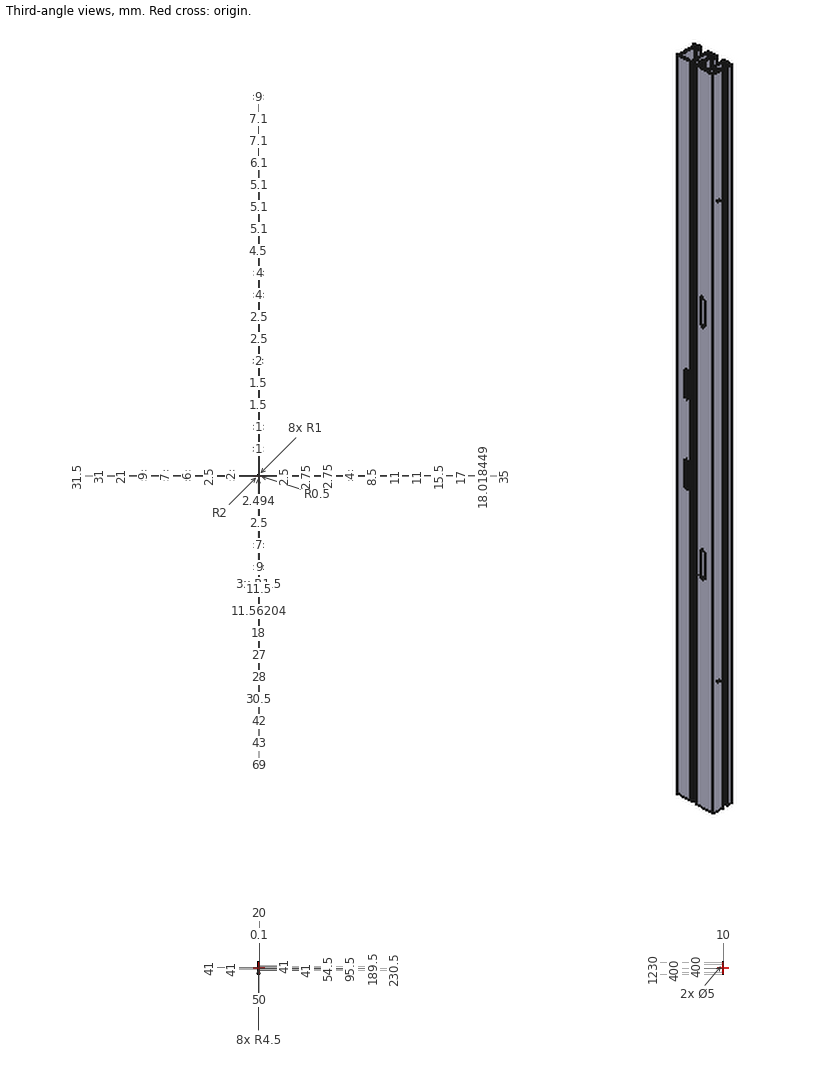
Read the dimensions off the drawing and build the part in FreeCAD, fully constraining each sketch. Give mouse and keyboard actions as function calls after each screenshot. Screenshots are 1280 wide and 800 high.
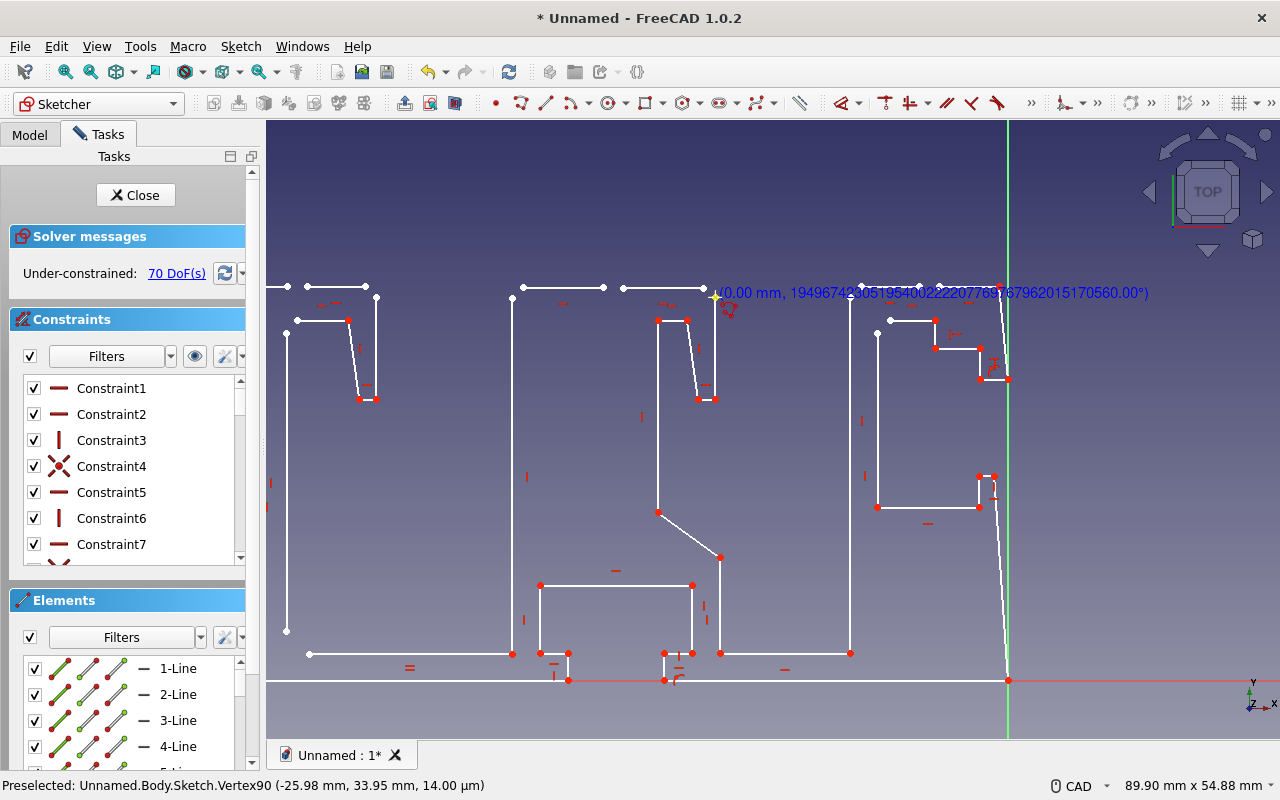
key(g)
key(3)
key(a)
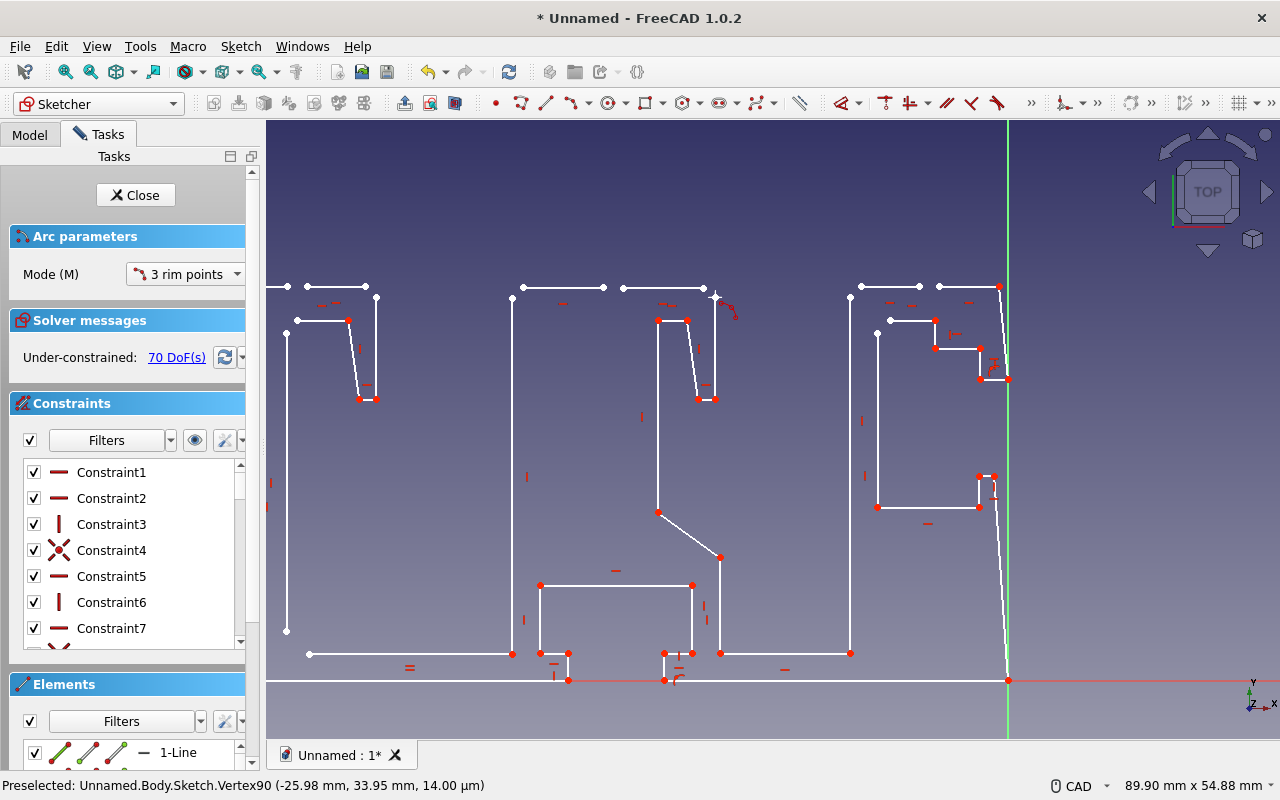
click(624, 288)
click(604, 288)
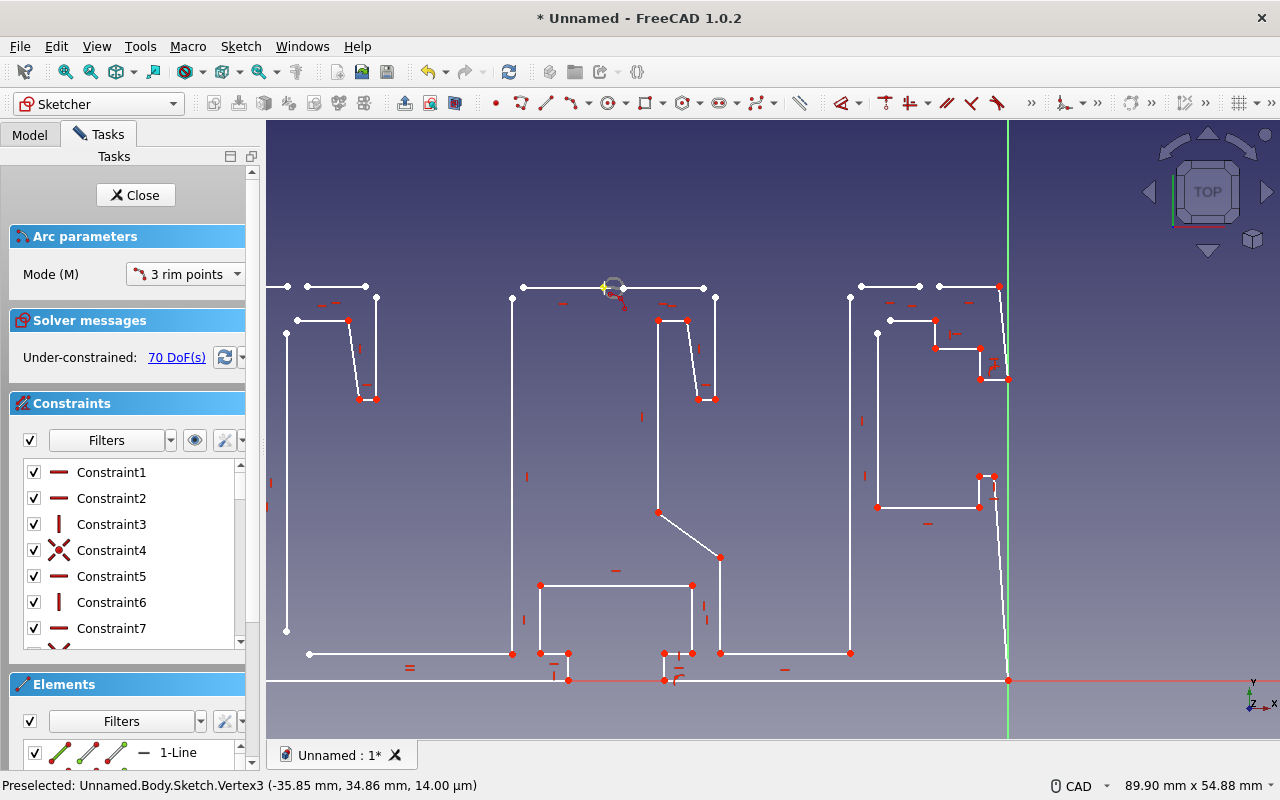
scroll(613, 289, up, 8)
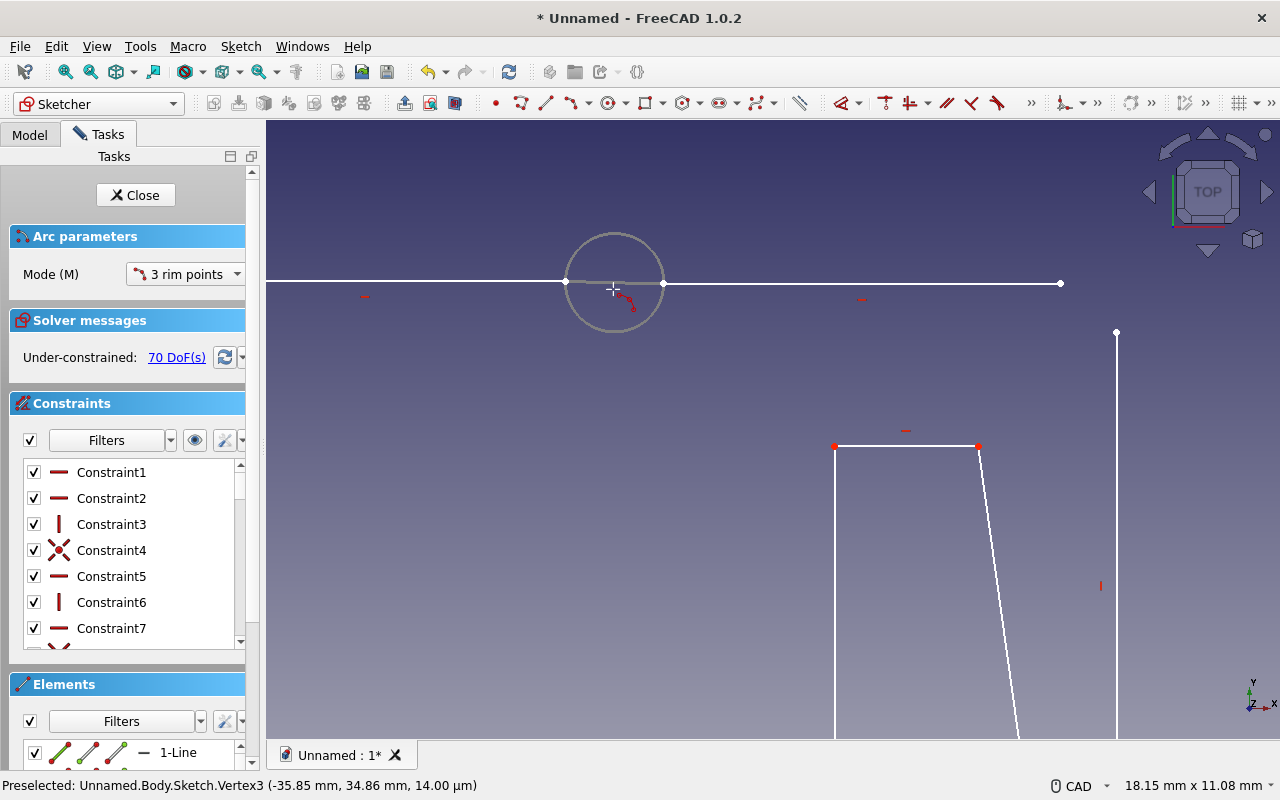
click(613, 290)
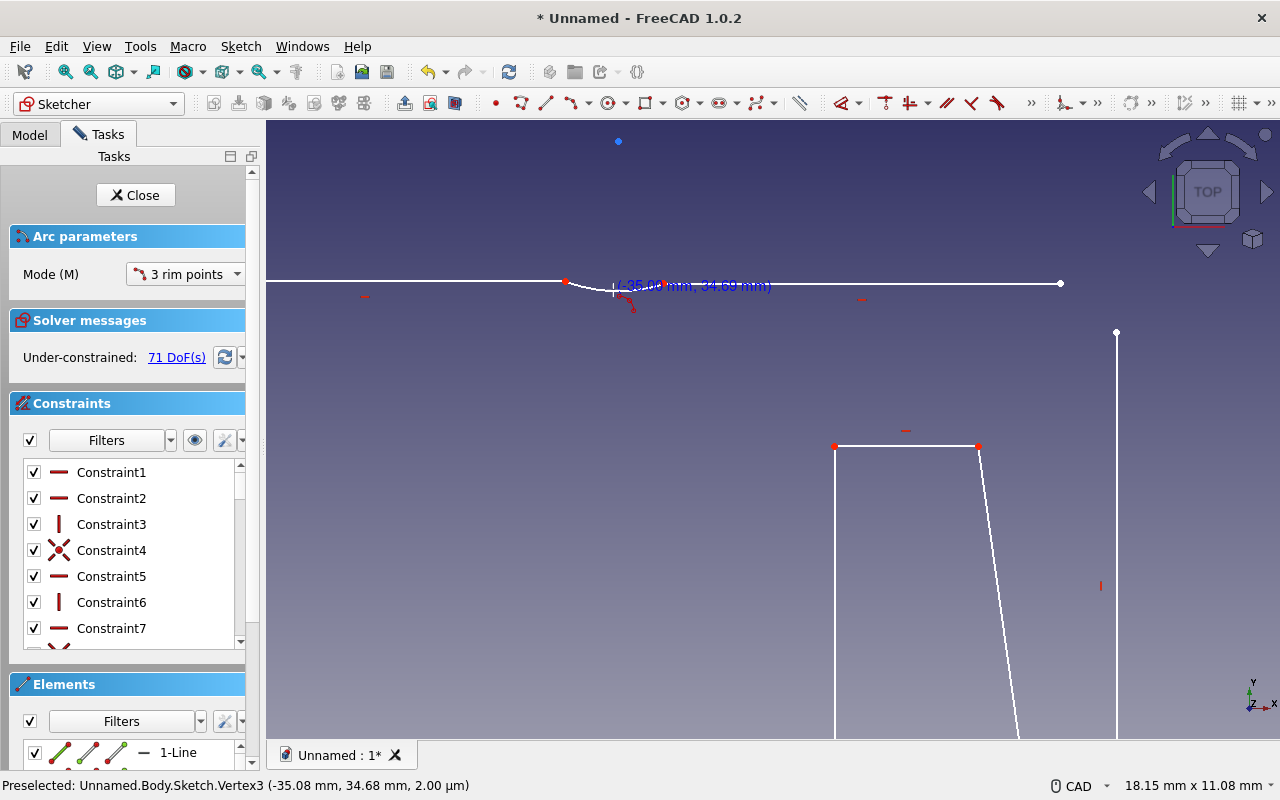
scroll(719, 301, down, 10)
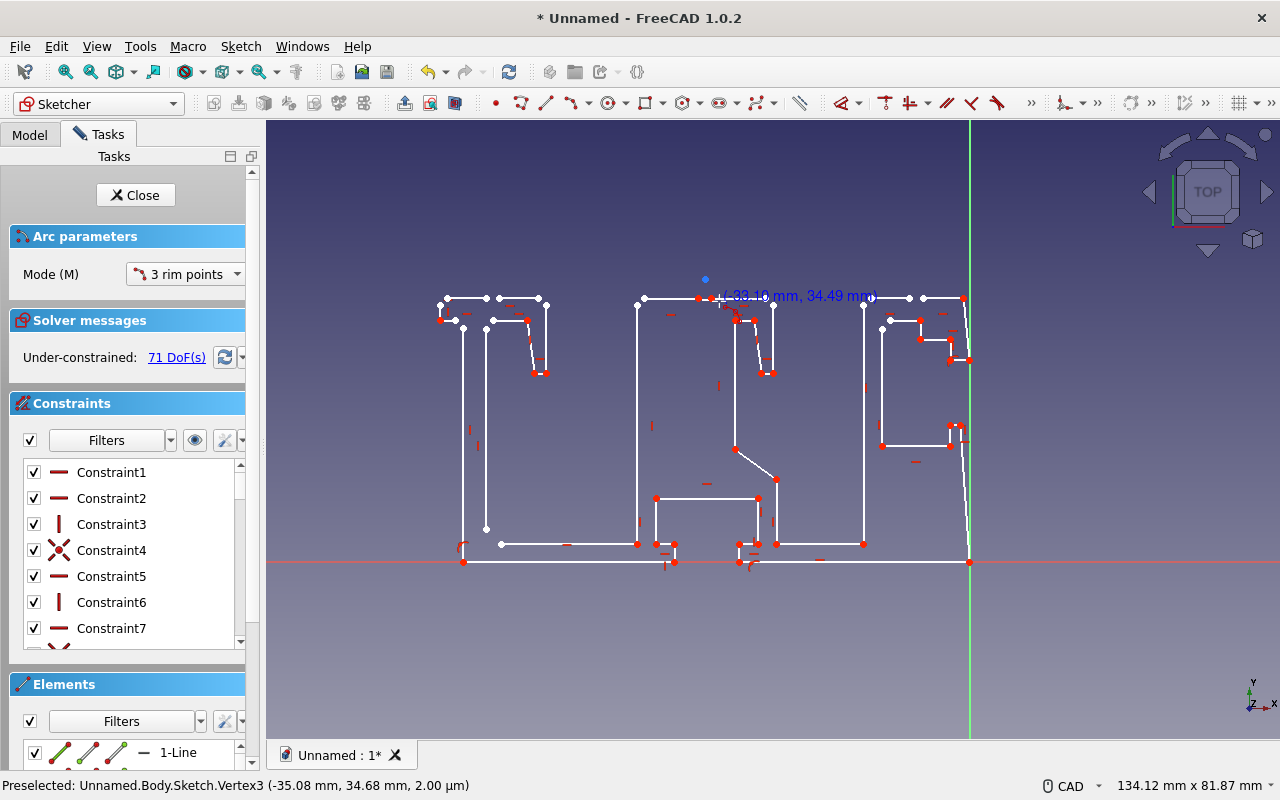
scroll(645, 298, up, 2)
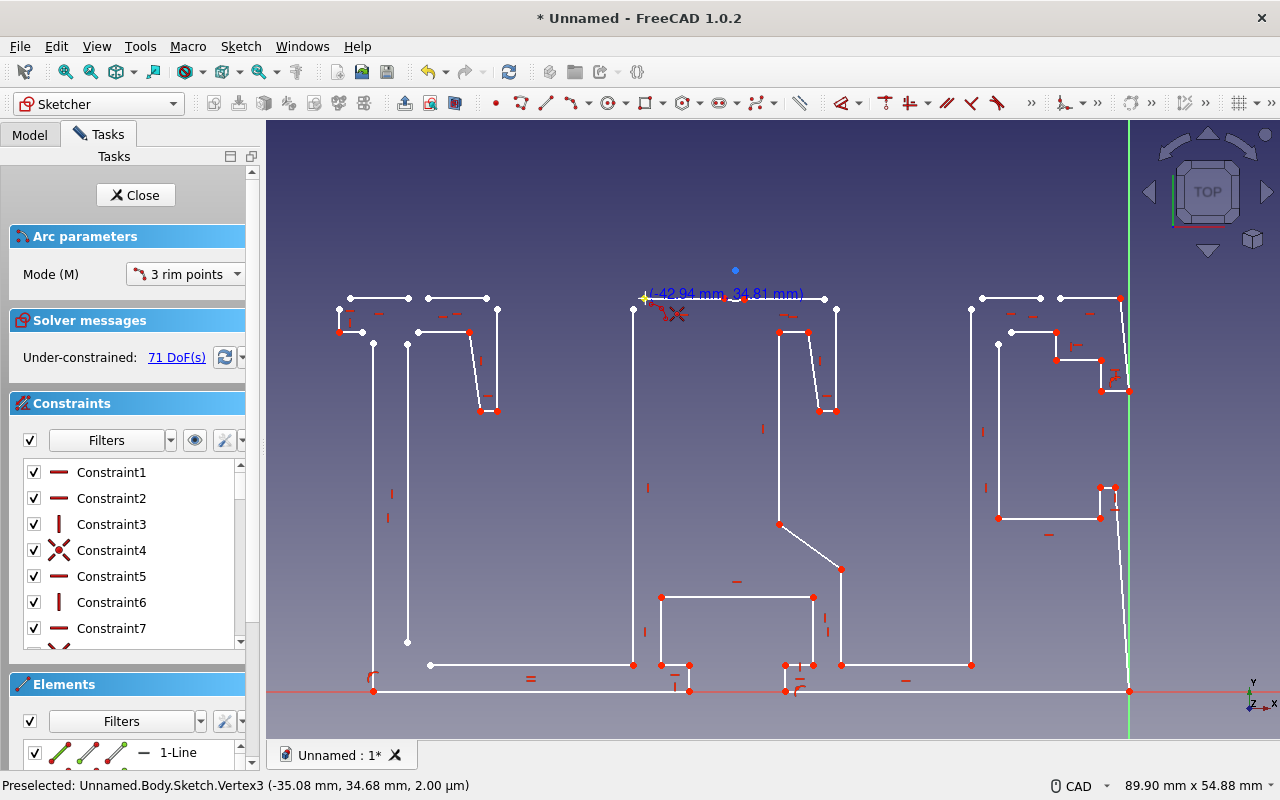
click(644, 299)
click(633, 310)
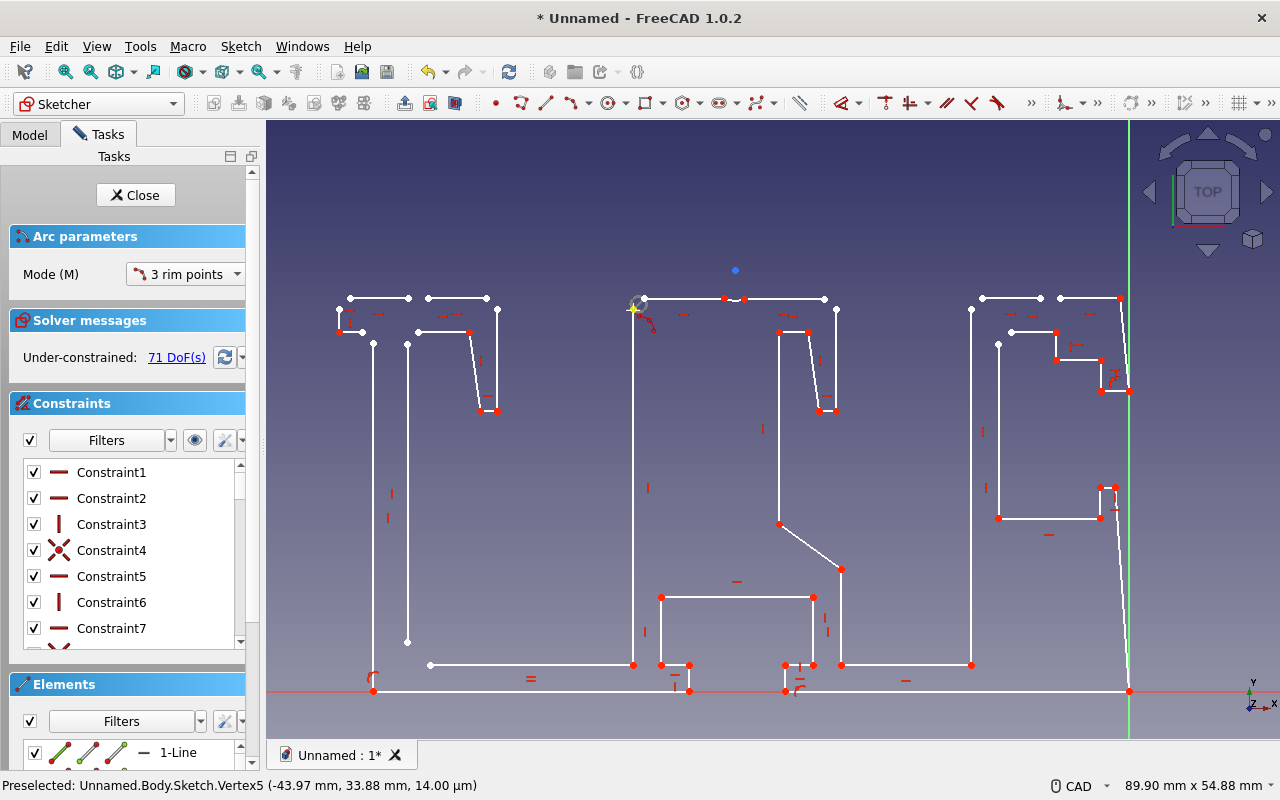
scroll(636, 300, up, 8)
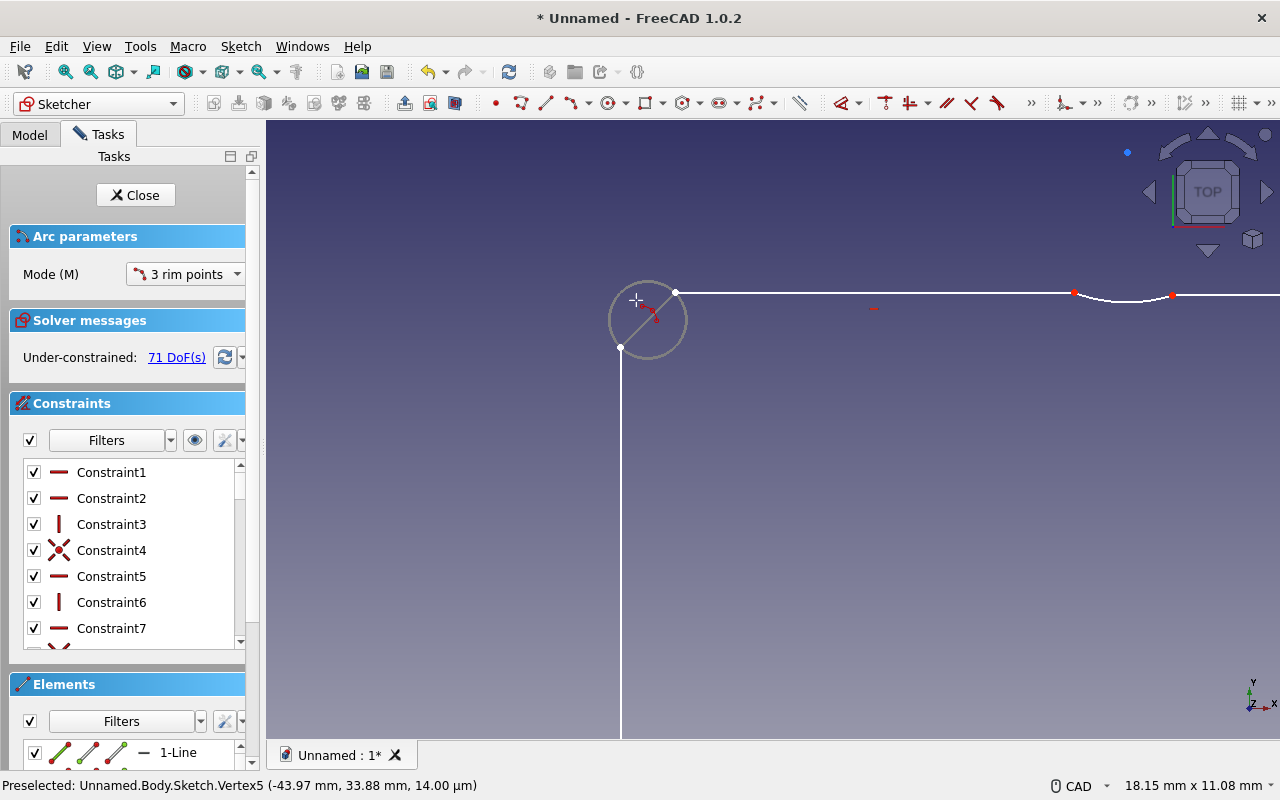
click(635, 301)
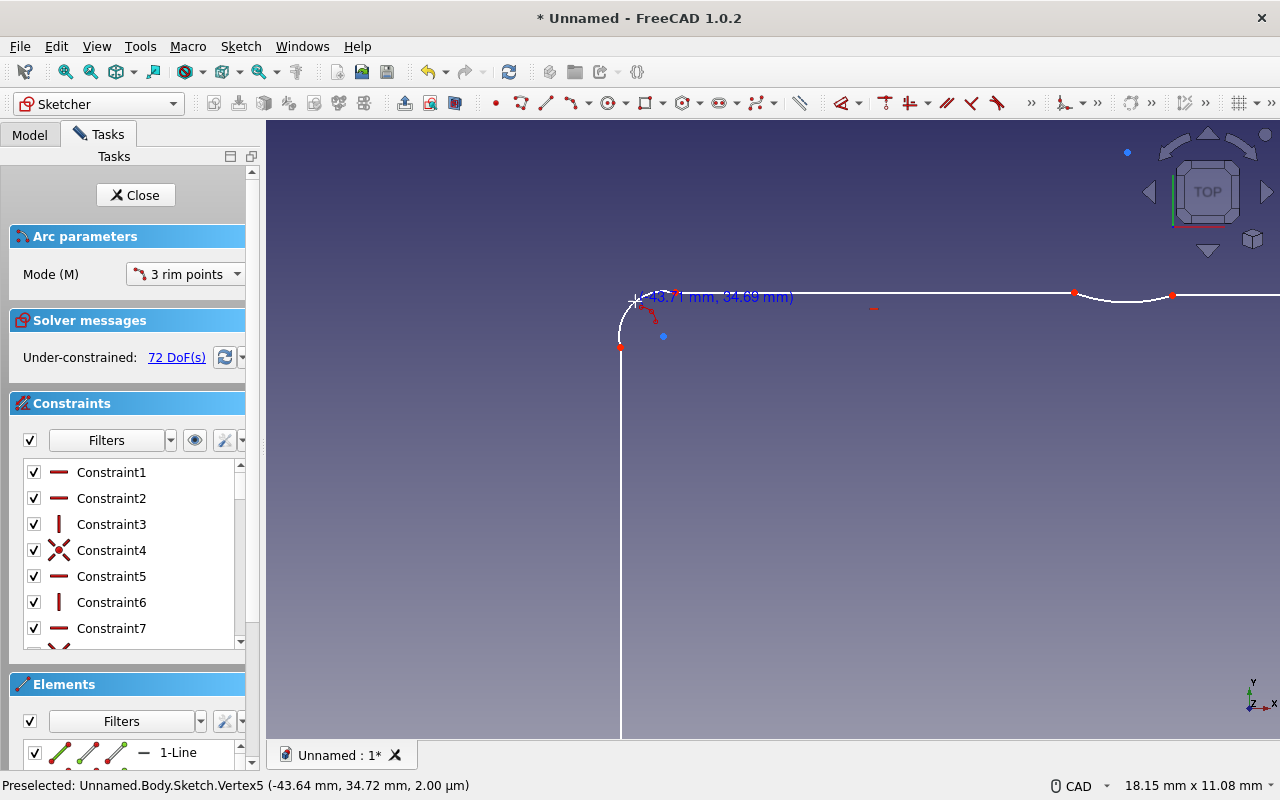
scroll(639, 299, down, 10)